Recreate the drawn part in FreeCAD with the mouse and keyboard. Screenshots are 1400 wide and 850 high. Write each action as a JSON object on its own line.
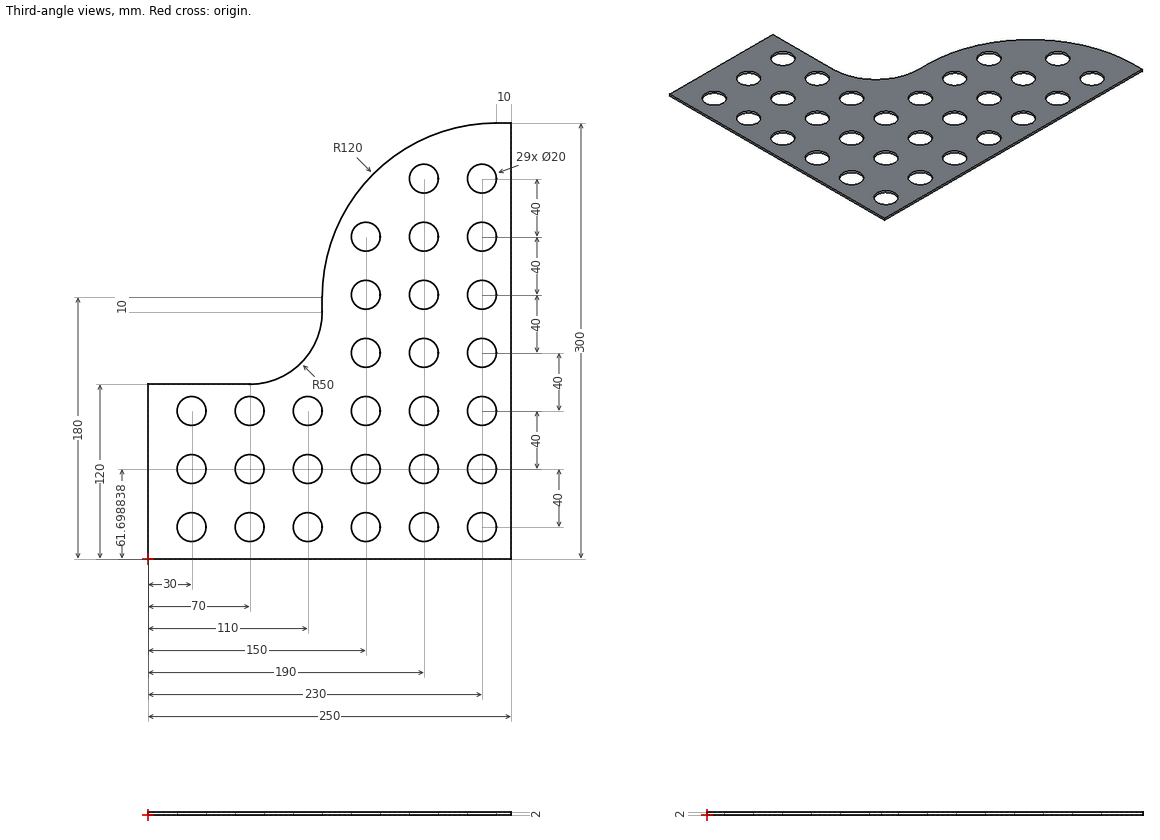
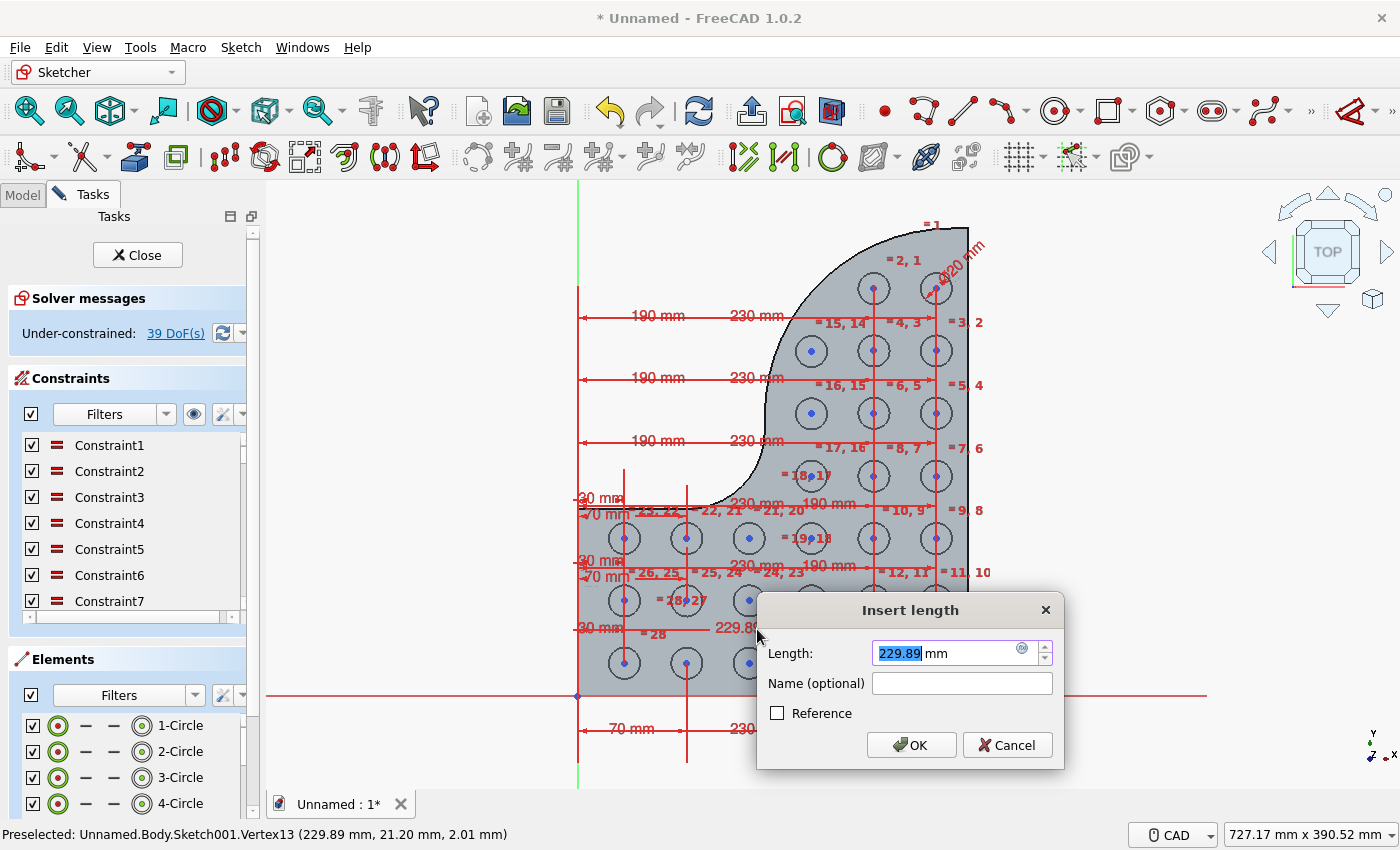
{"action": "type", "text": "230"}
{"action": "key", "text": "Return"}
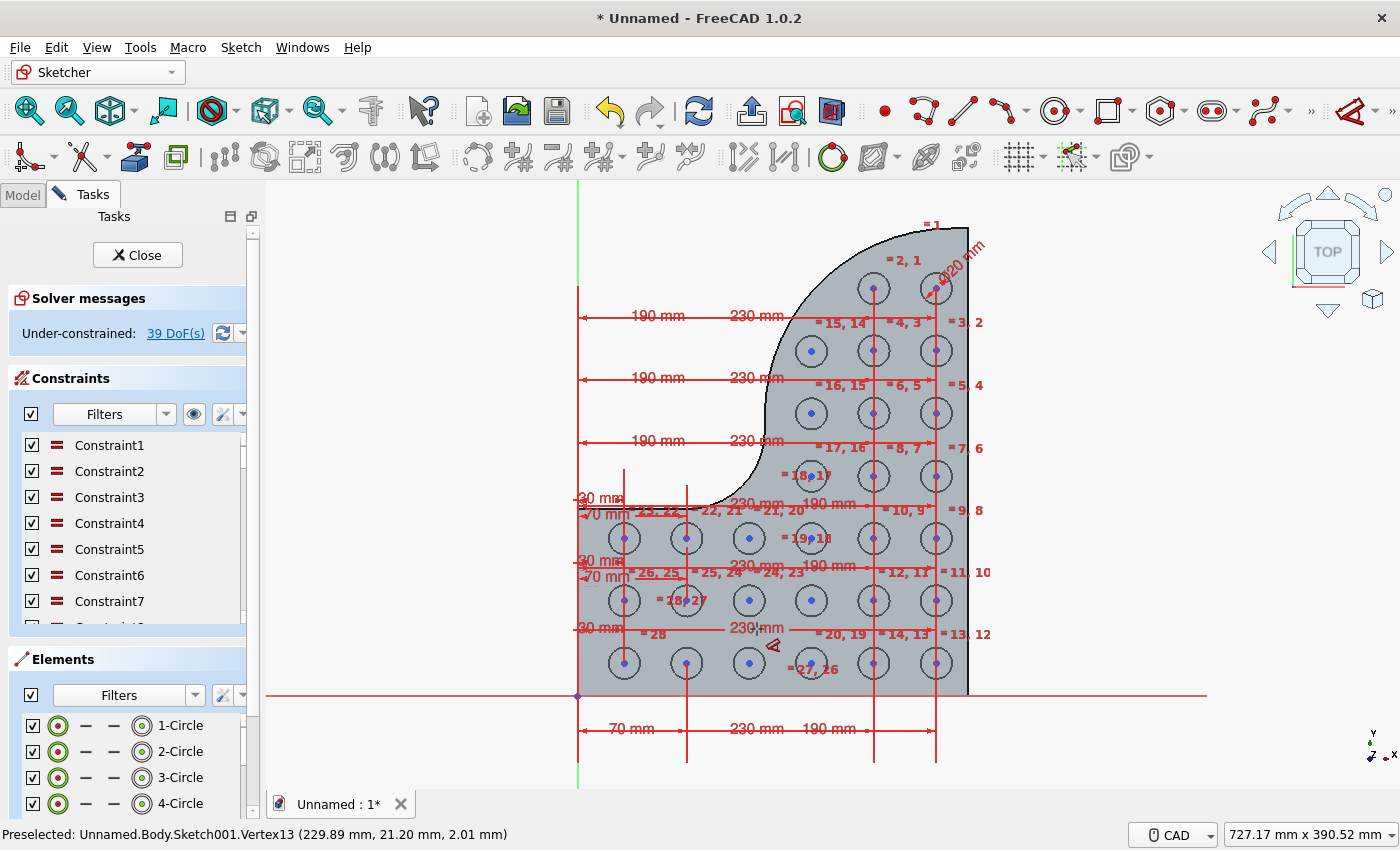
{"action": "left_click", "coordinate": [874, 663]}
{"action": "left_click", "coordinate": [829, 629]}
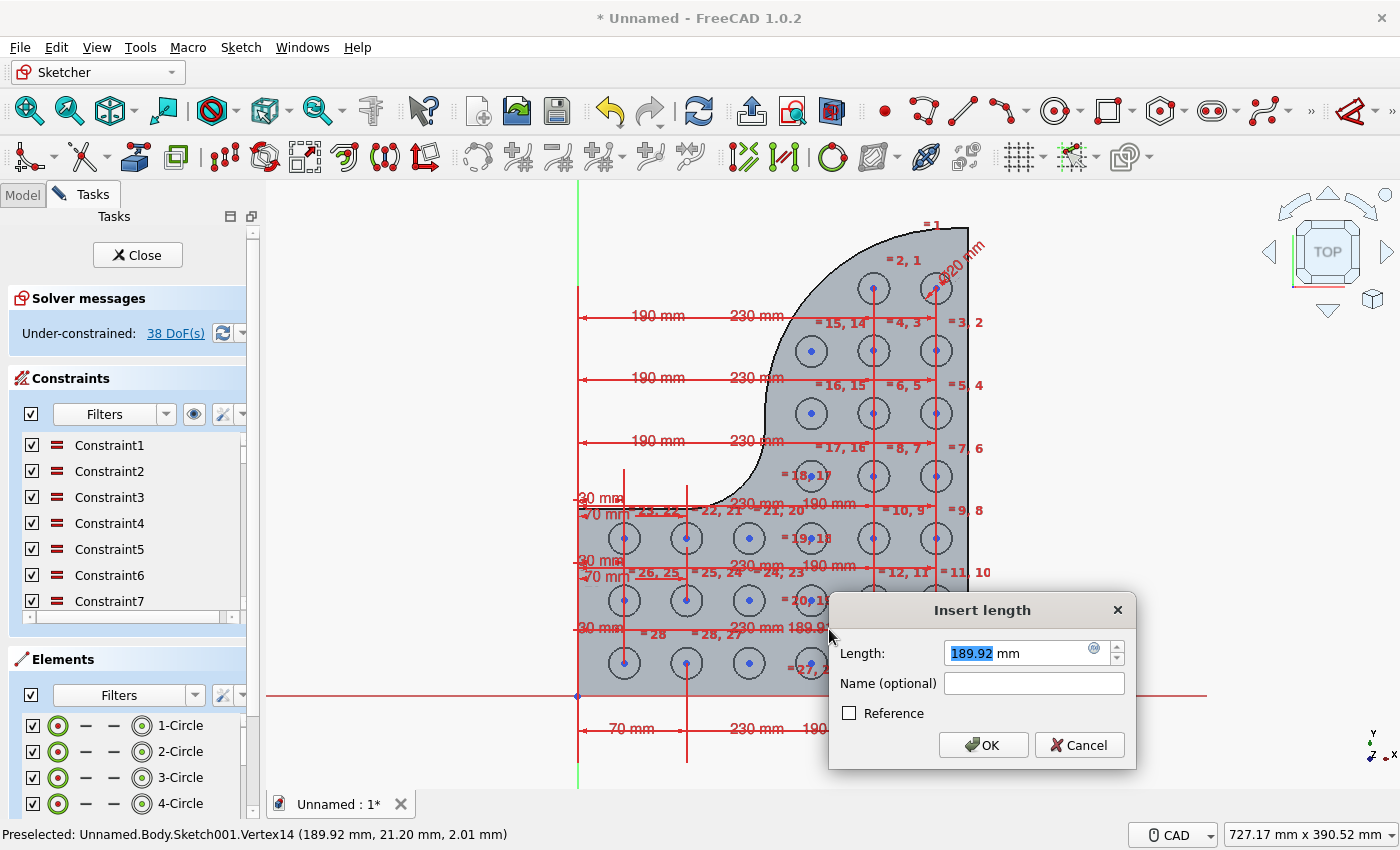
{"action": "type", "text": "190"}
{"action": "key", "text": "Return"}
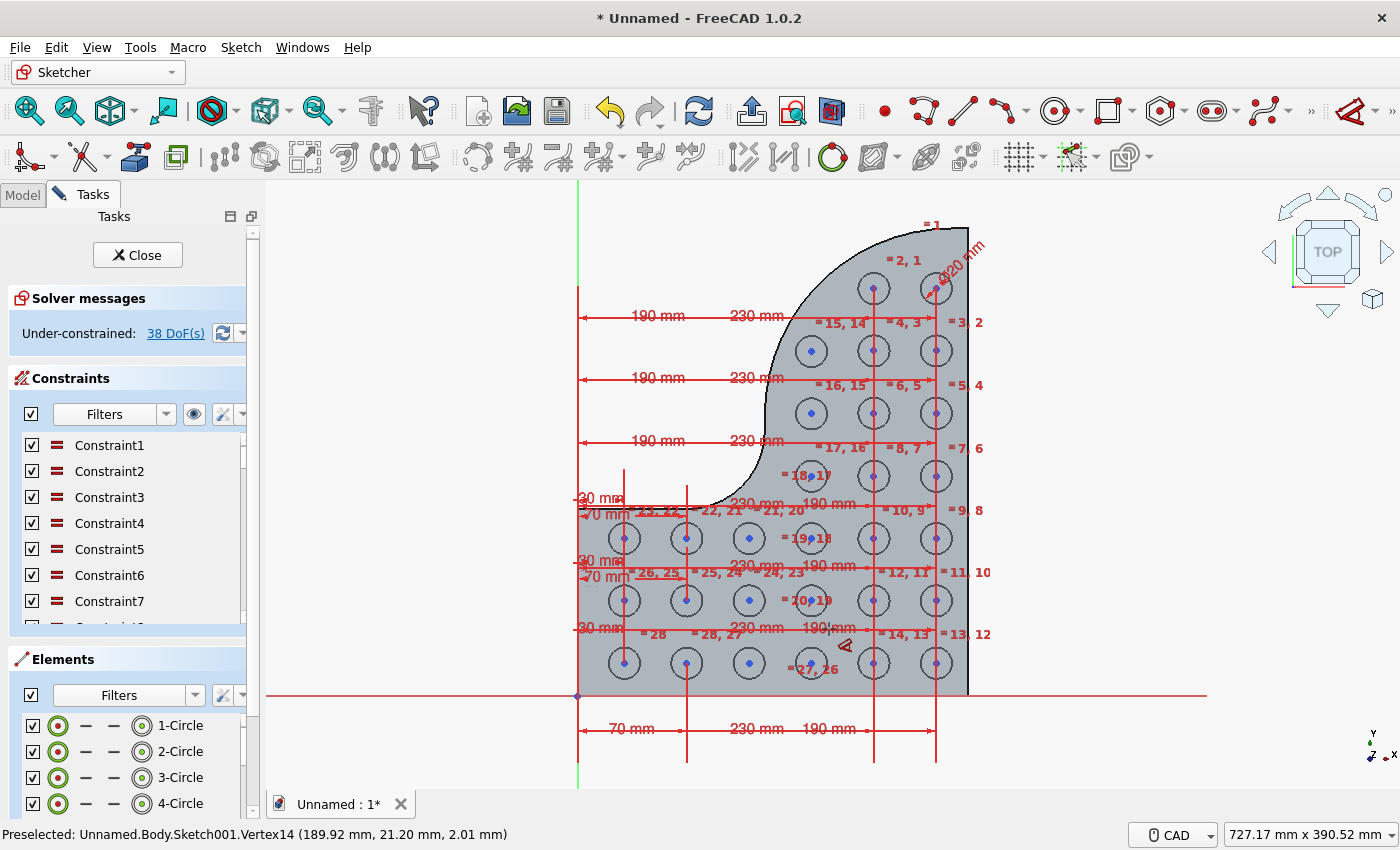
{"action": "left_click", "coordinate": [812, 352]}
{"action": "left_click", "coordinate": [695, 754]}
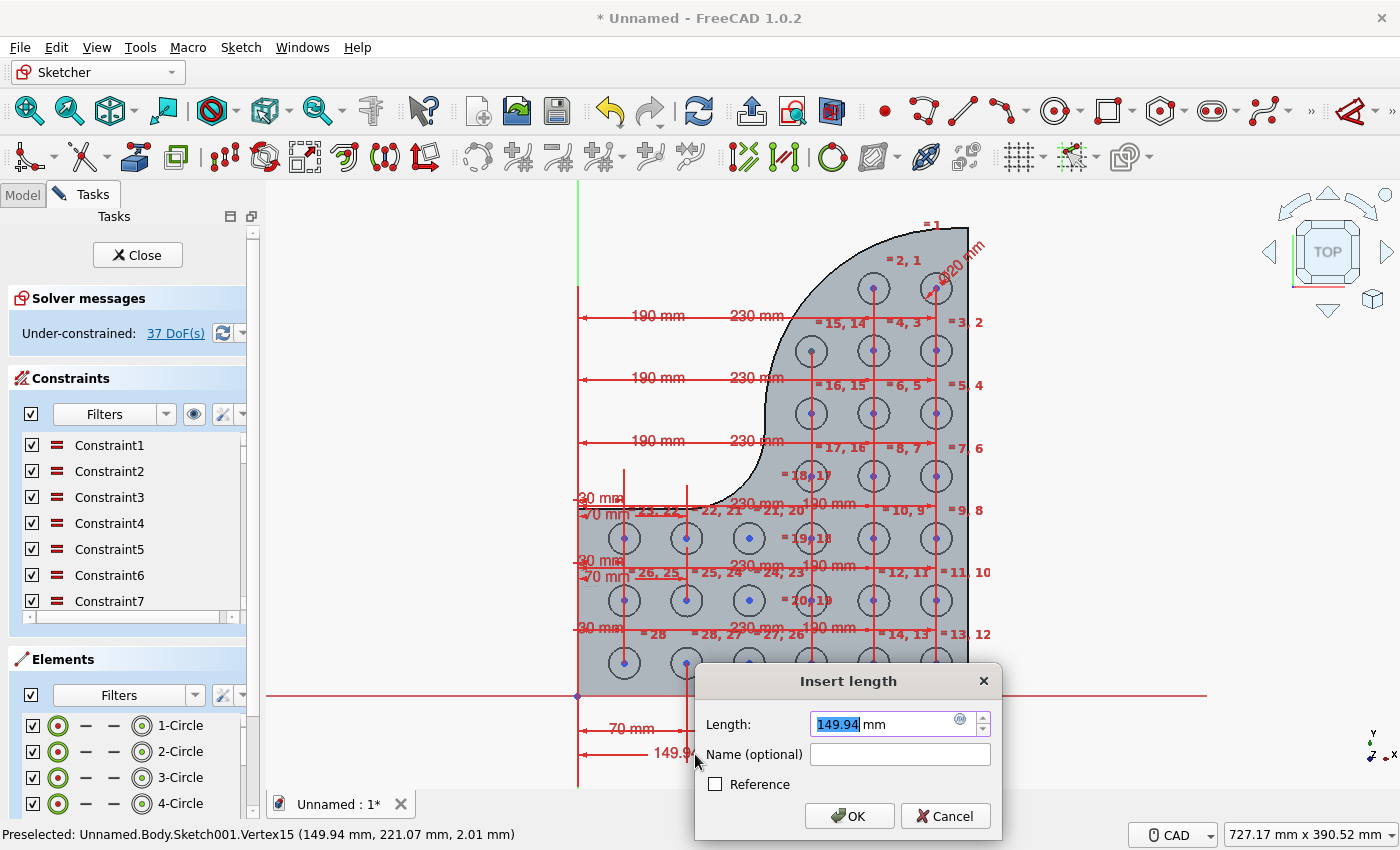
{"action": "type", "text": "150"}
{"action": "key", "text": "Return"}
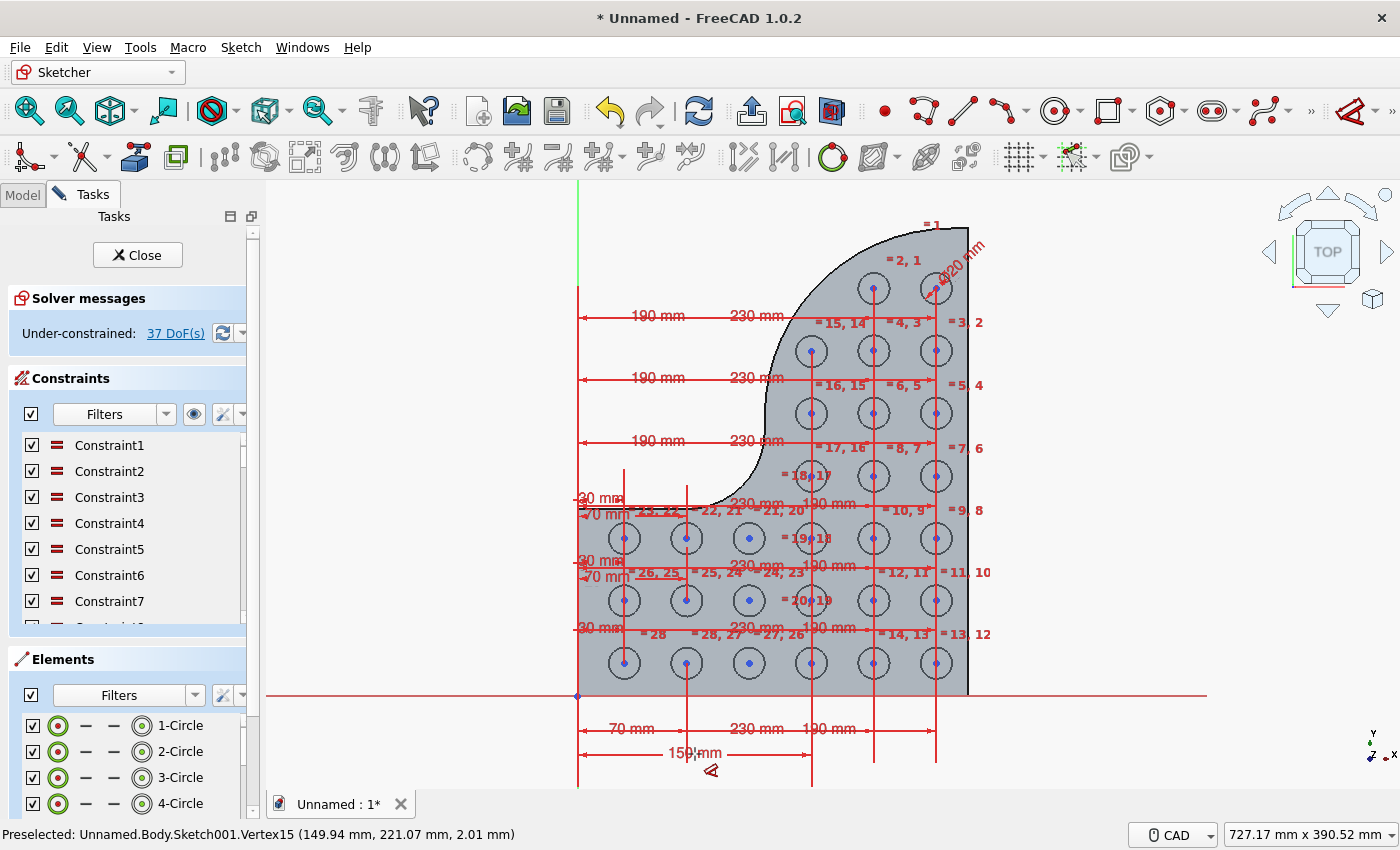
{"action": "left_click", "coordinate": [812, 414]}
{"action": "left_click", "coordinate": [613, 754]}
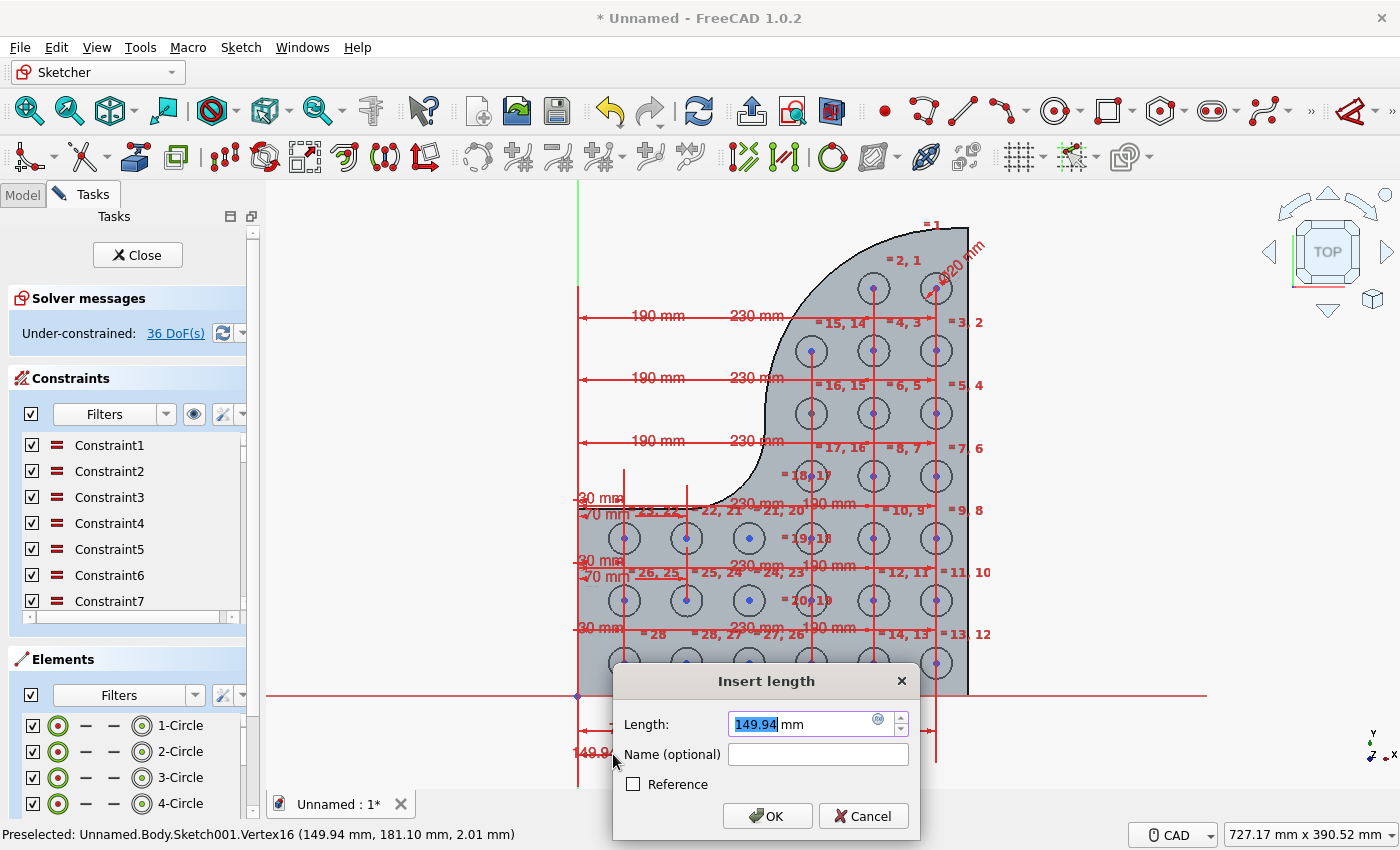
{"action": "type", "text": "150"}
{"action": "key", "text": "Return"}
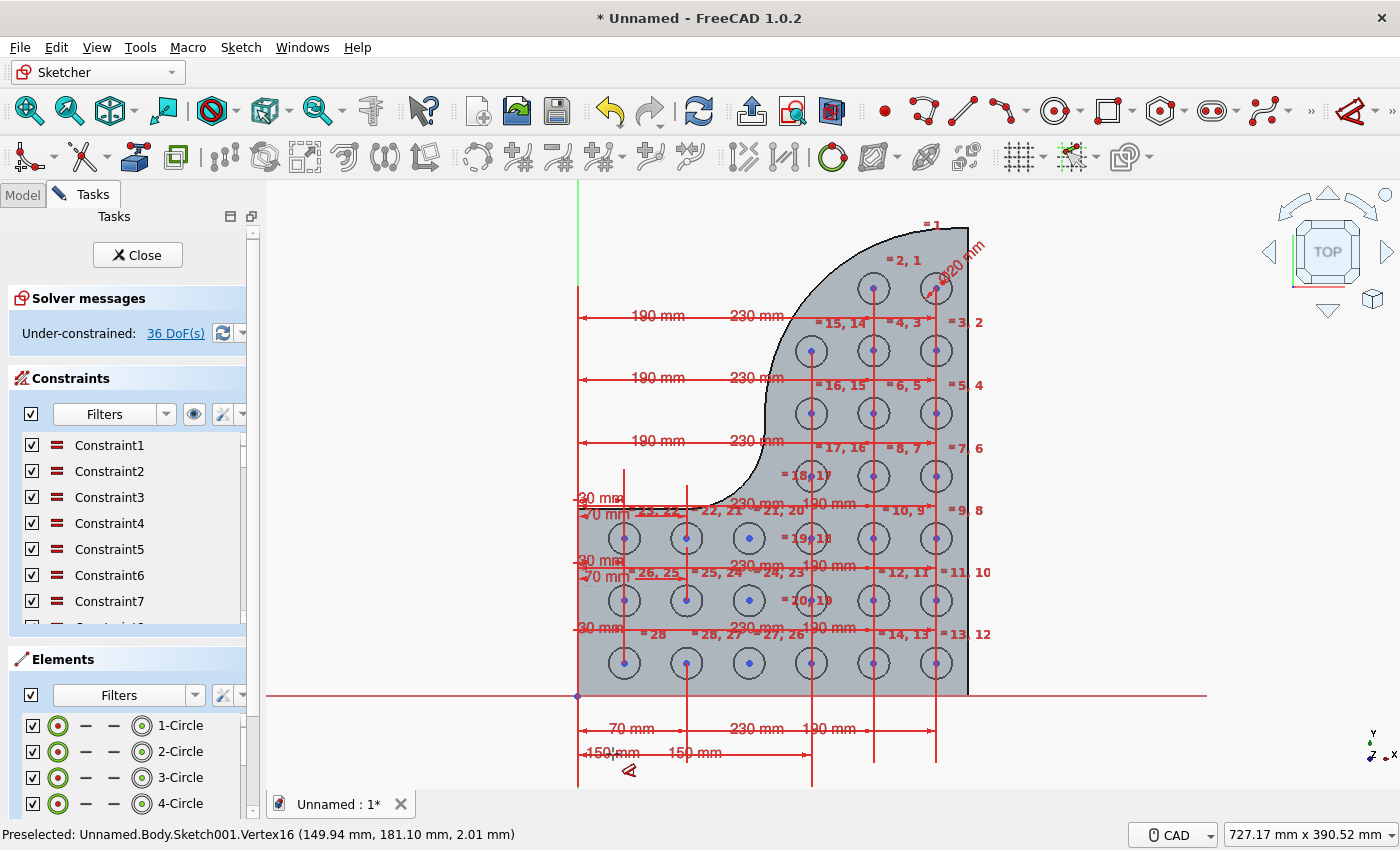
{"action": "left_click", "coordinate": [812, 476]}
{"action": "left_click", "coordinate": [776, 754]}